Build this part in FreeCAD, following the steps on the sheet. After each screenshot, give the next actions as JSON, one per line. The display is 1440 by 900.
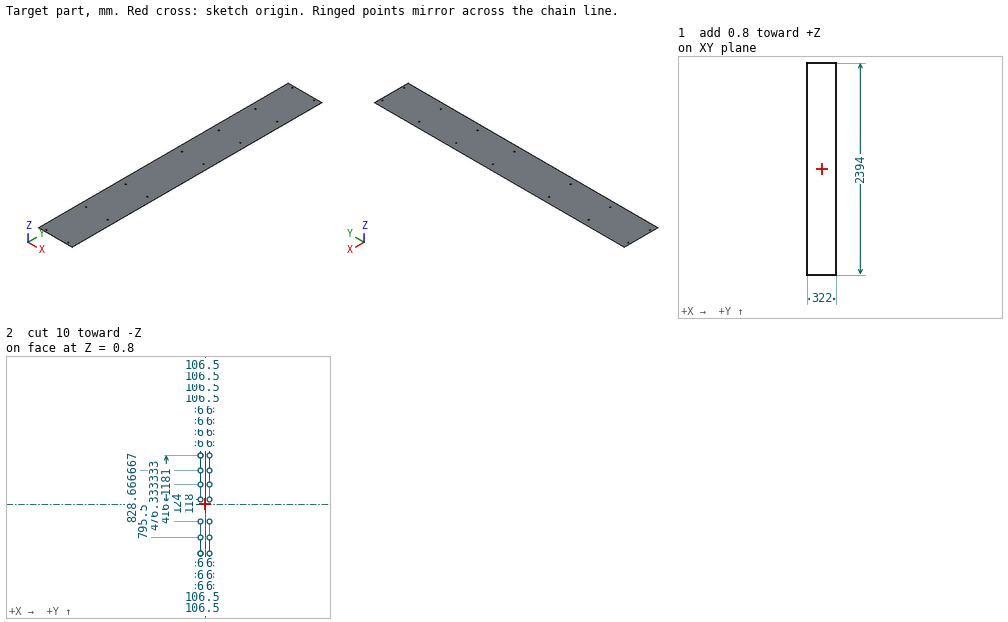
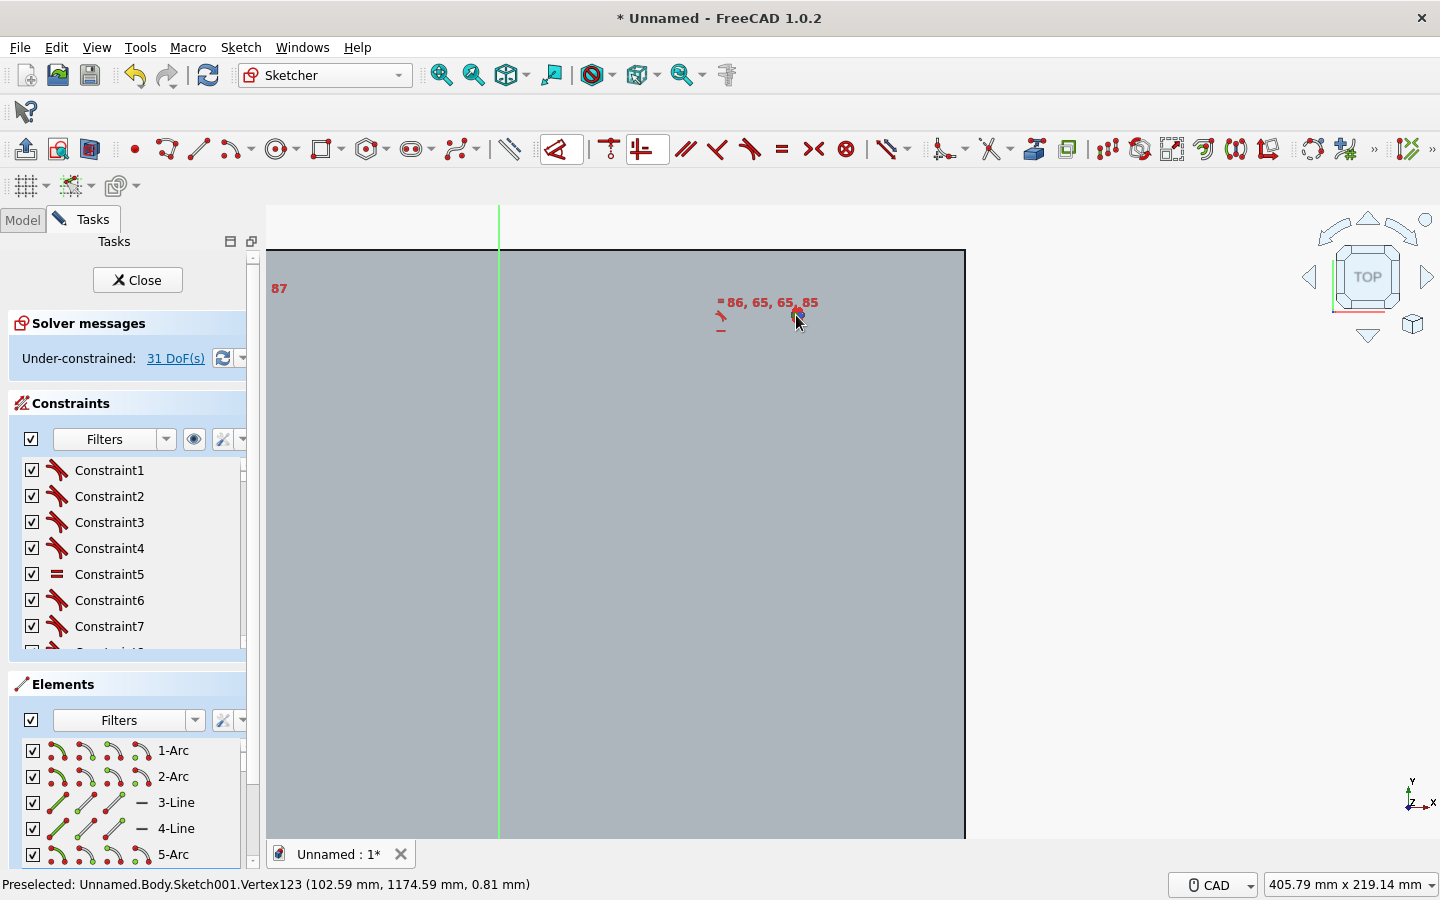
{"action": "left_click", "coordinate": [499, 770]}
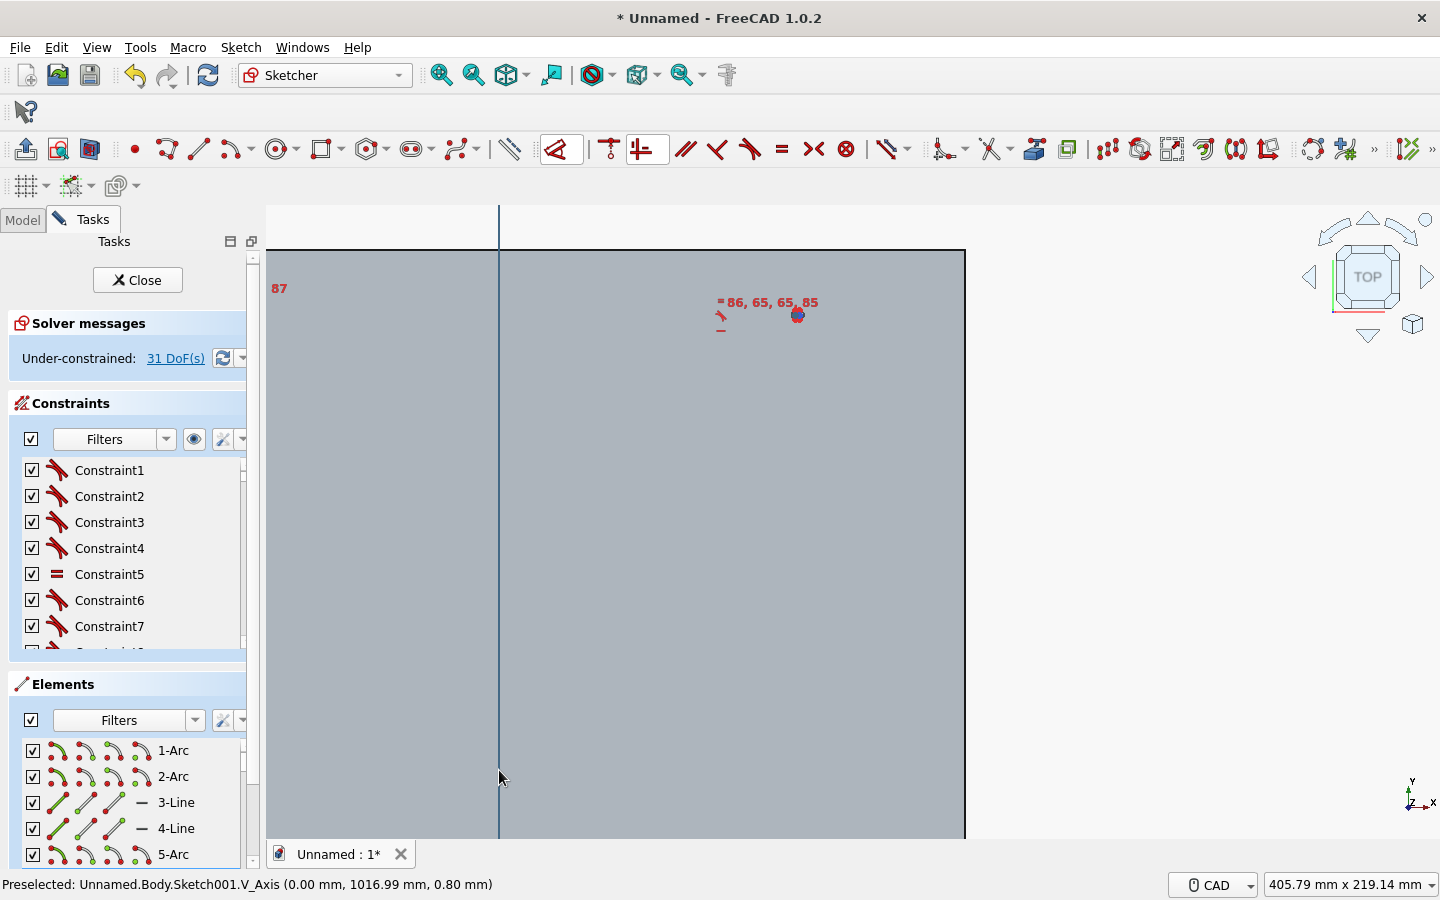
{"action": "key", "text": "s"}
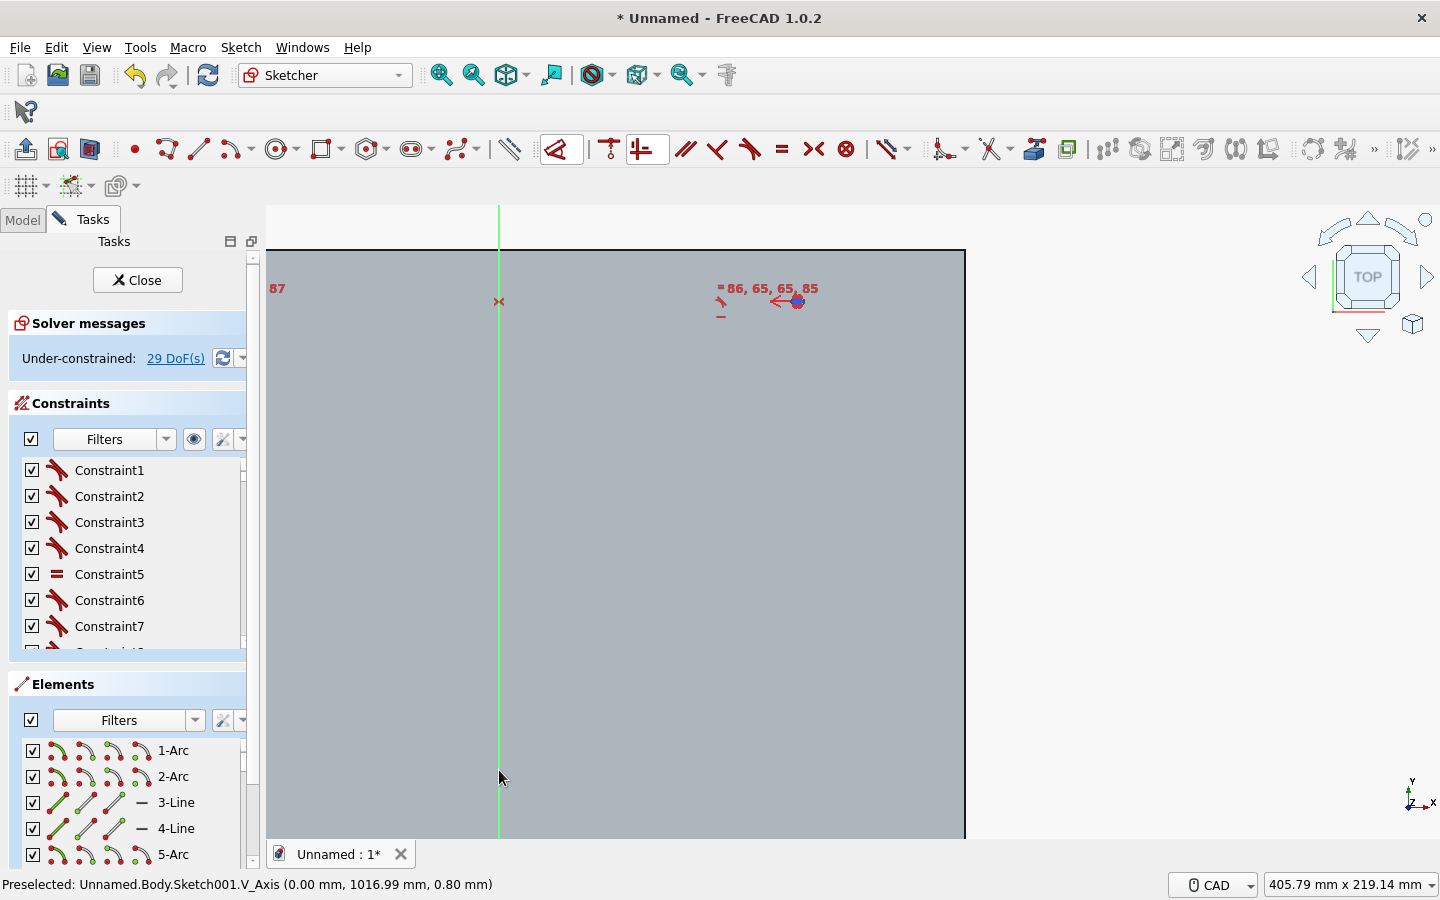
{"action": "scroll", "coordinate": [803, 315], "scroll_direction": "down", "scroll_amount": 14}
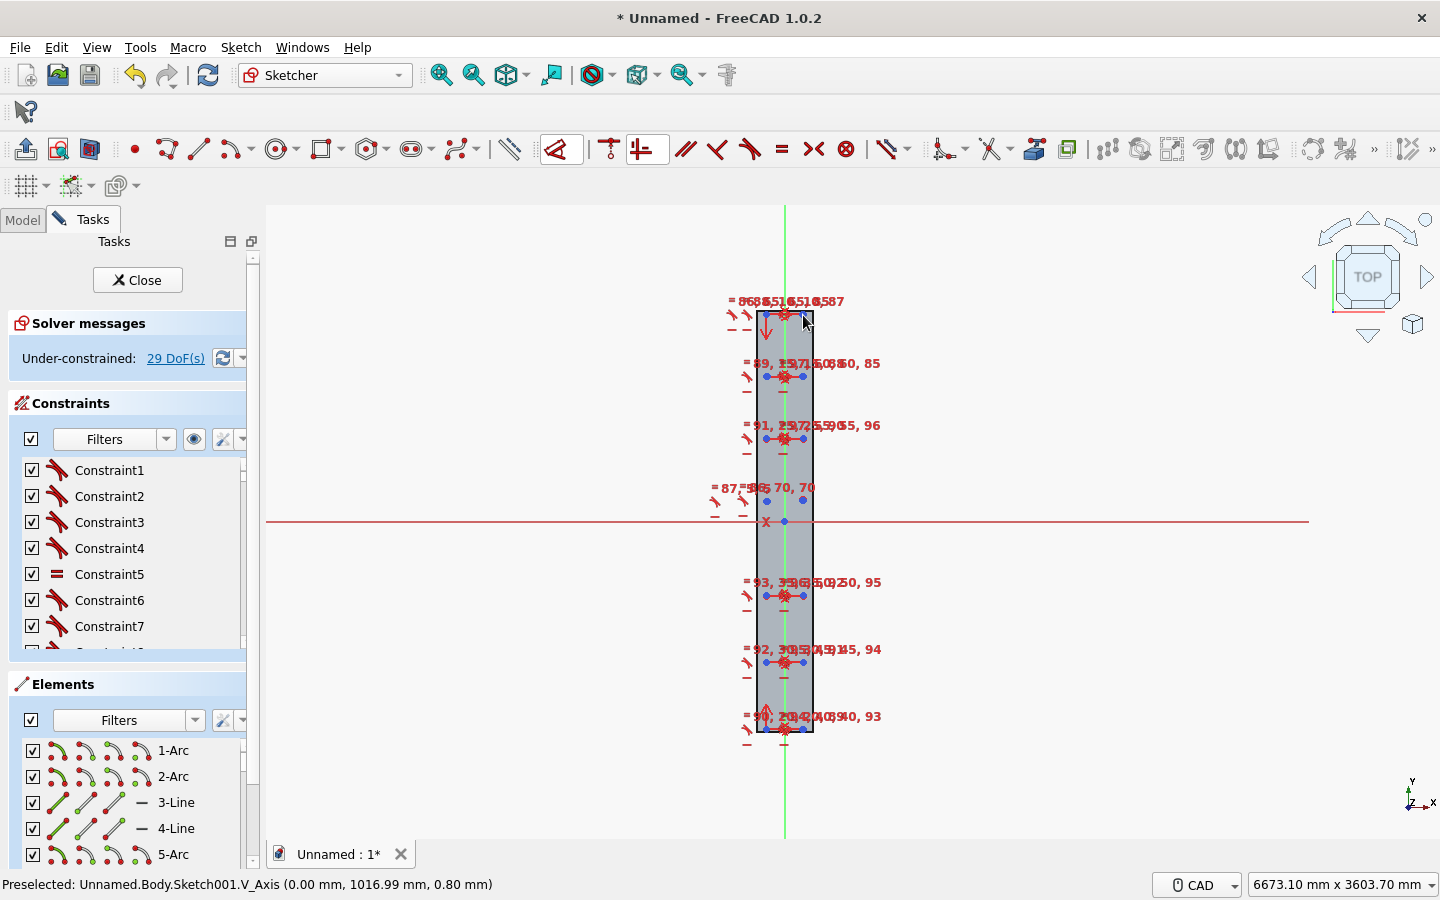
{"action": "scroll", "coordinate": [767, 502], "scroll_direction": "up", "scroll_amount": 14}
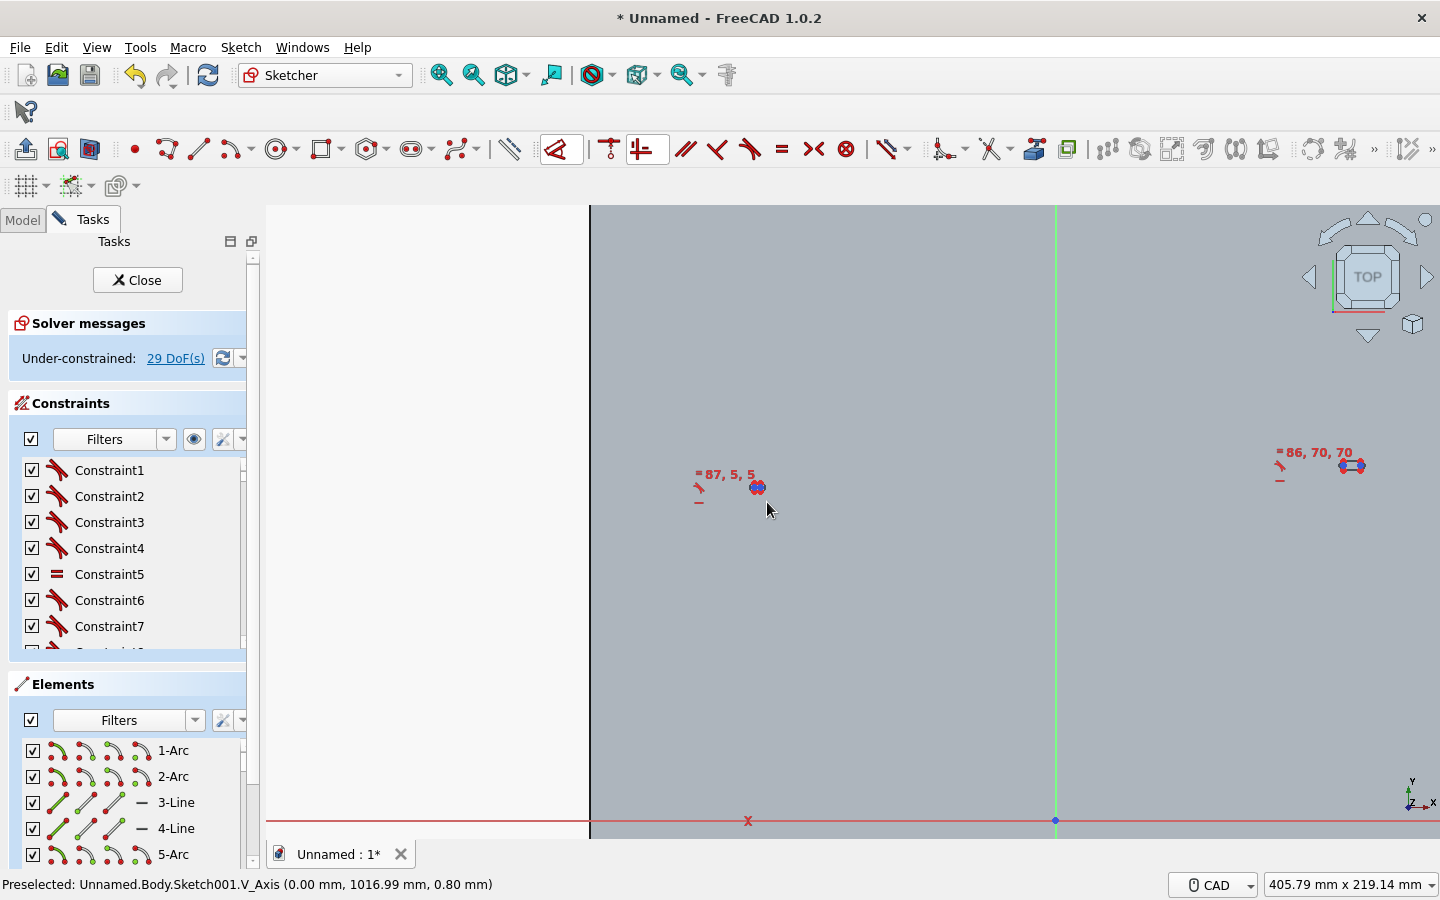
{"action": "left_click", "coordinate": [761, 488]}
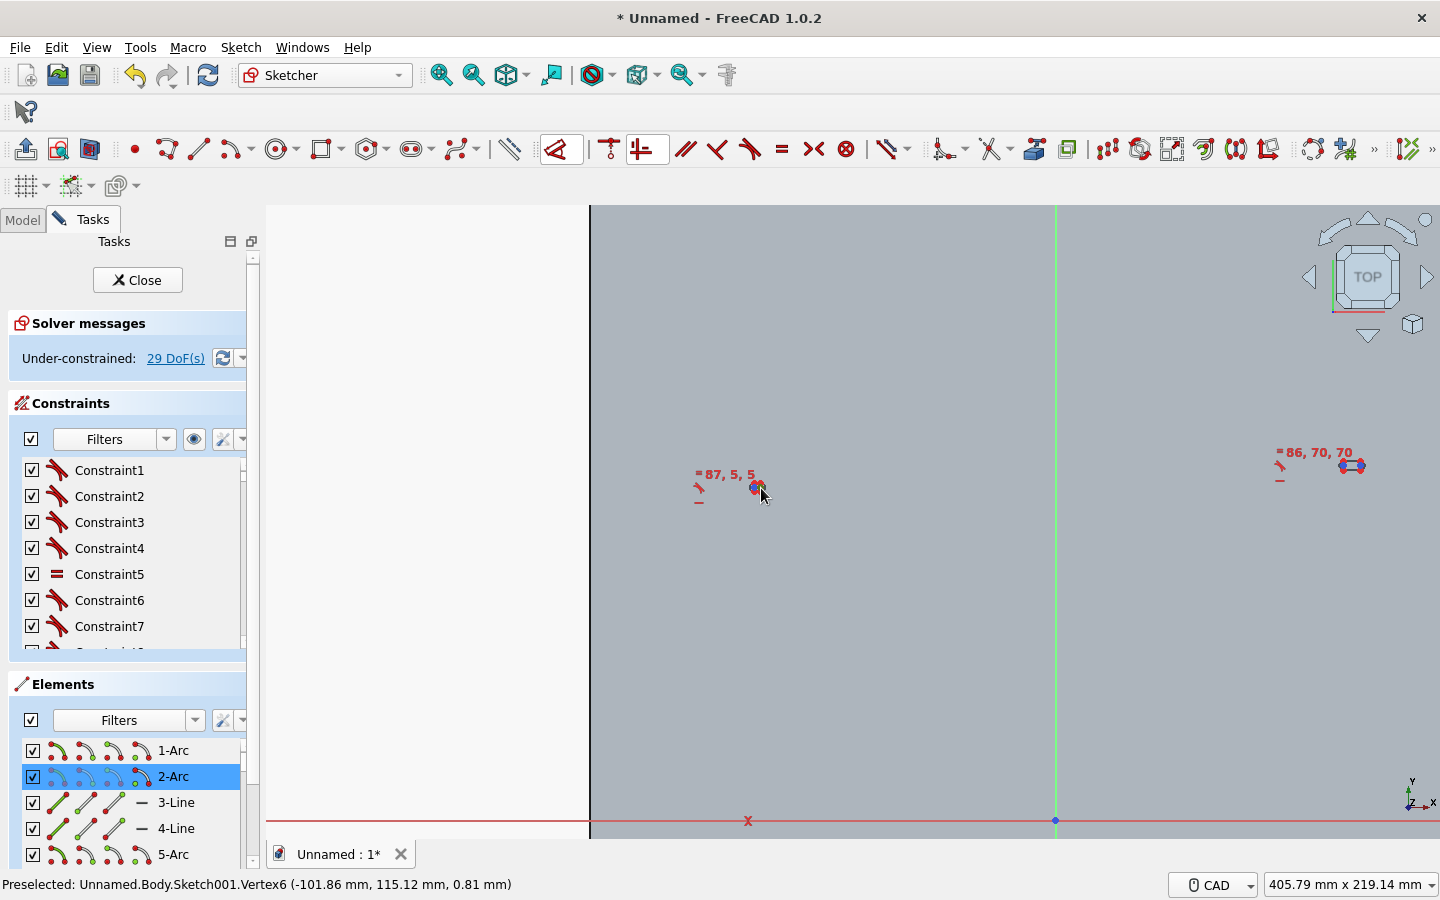
{"action": "scroll", "coordinate": [767, 503], "scroll_direction": "down", "scroll_amount": 14}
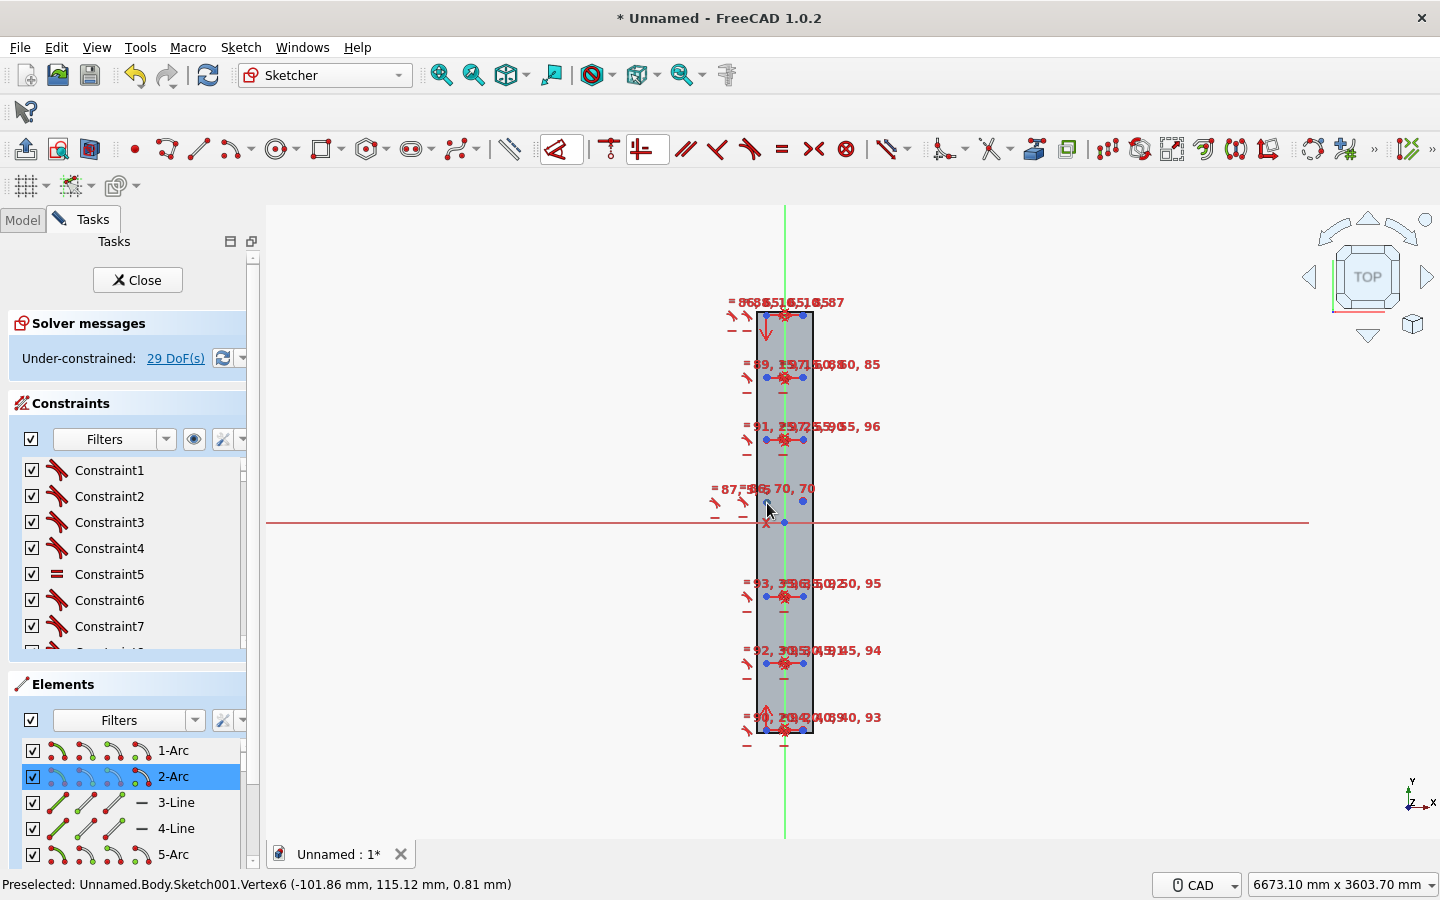
{"action": "scroll", "coordinate": [802, 501], "scroll_direction": "up", "scroll_amount": 14}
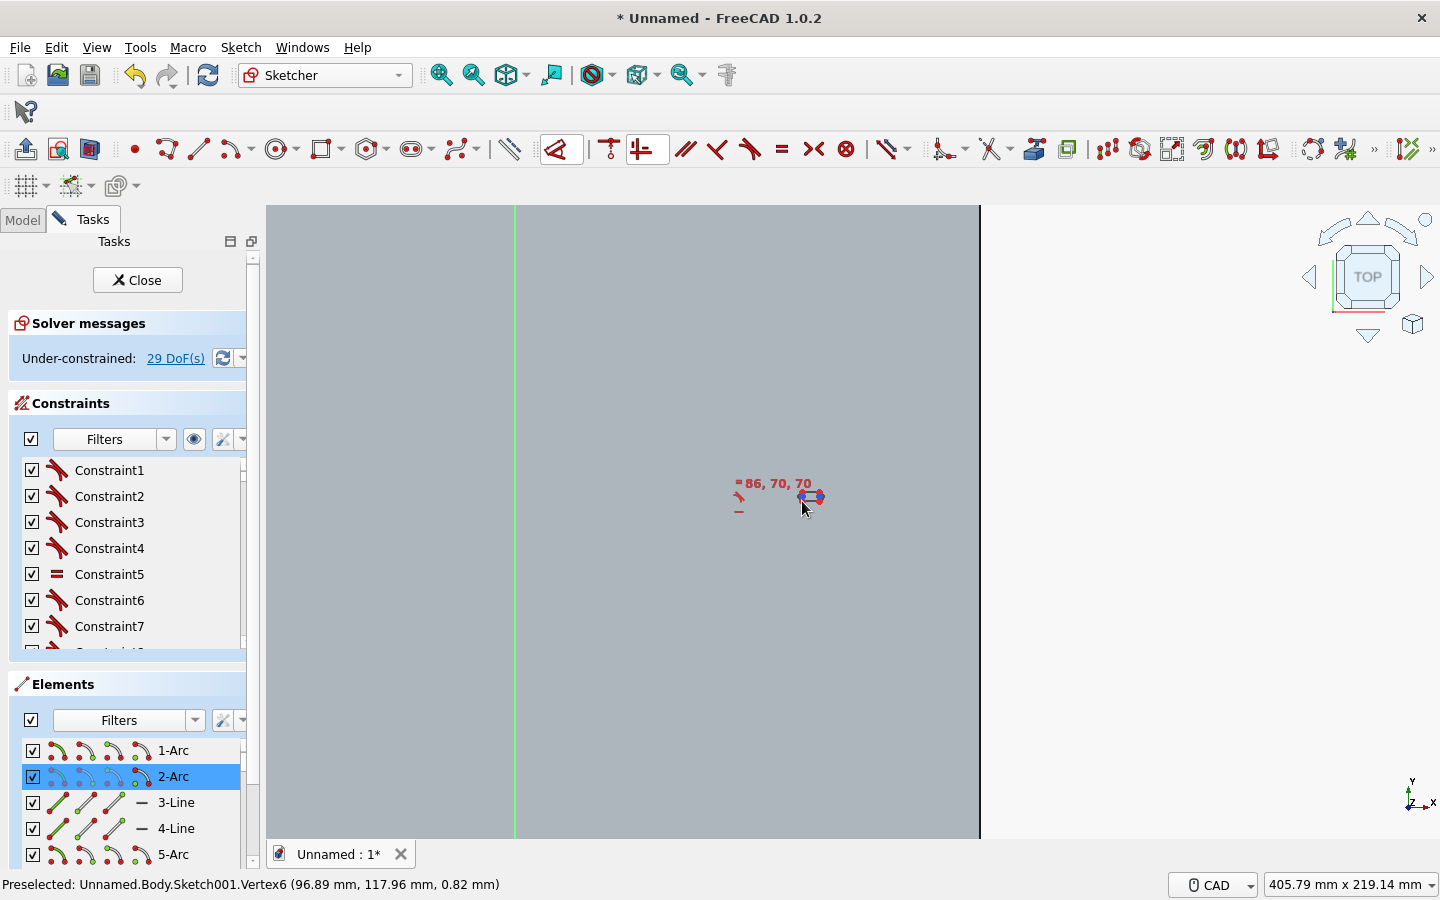
{"action": "scroll", "coordinate": [803, 497], "scroll_direction": "up", "scroll_amount": 4}